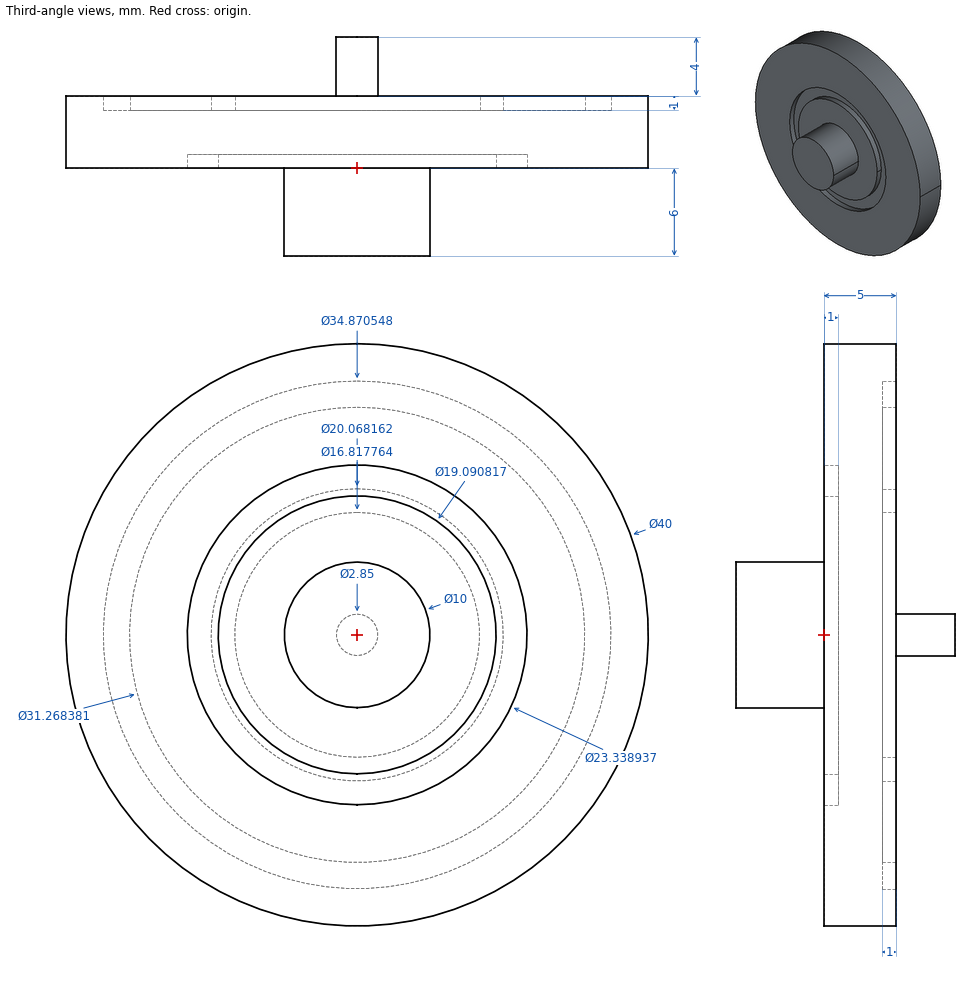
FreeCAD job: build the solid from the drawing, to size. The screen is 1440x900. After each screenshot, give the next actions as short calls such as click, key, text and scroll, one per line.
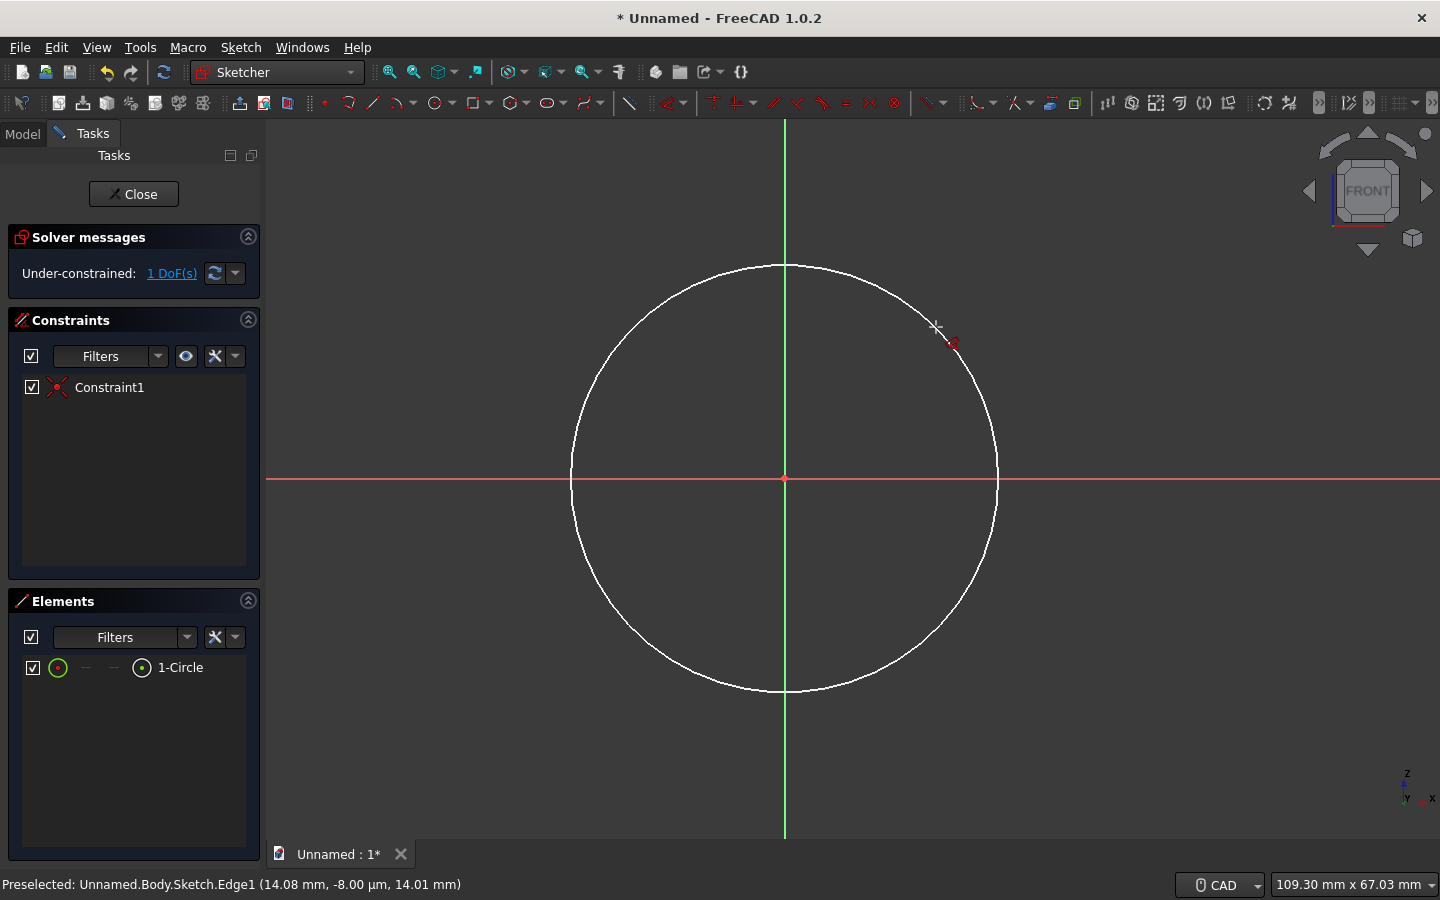
click(935, 327)
click(958, 304)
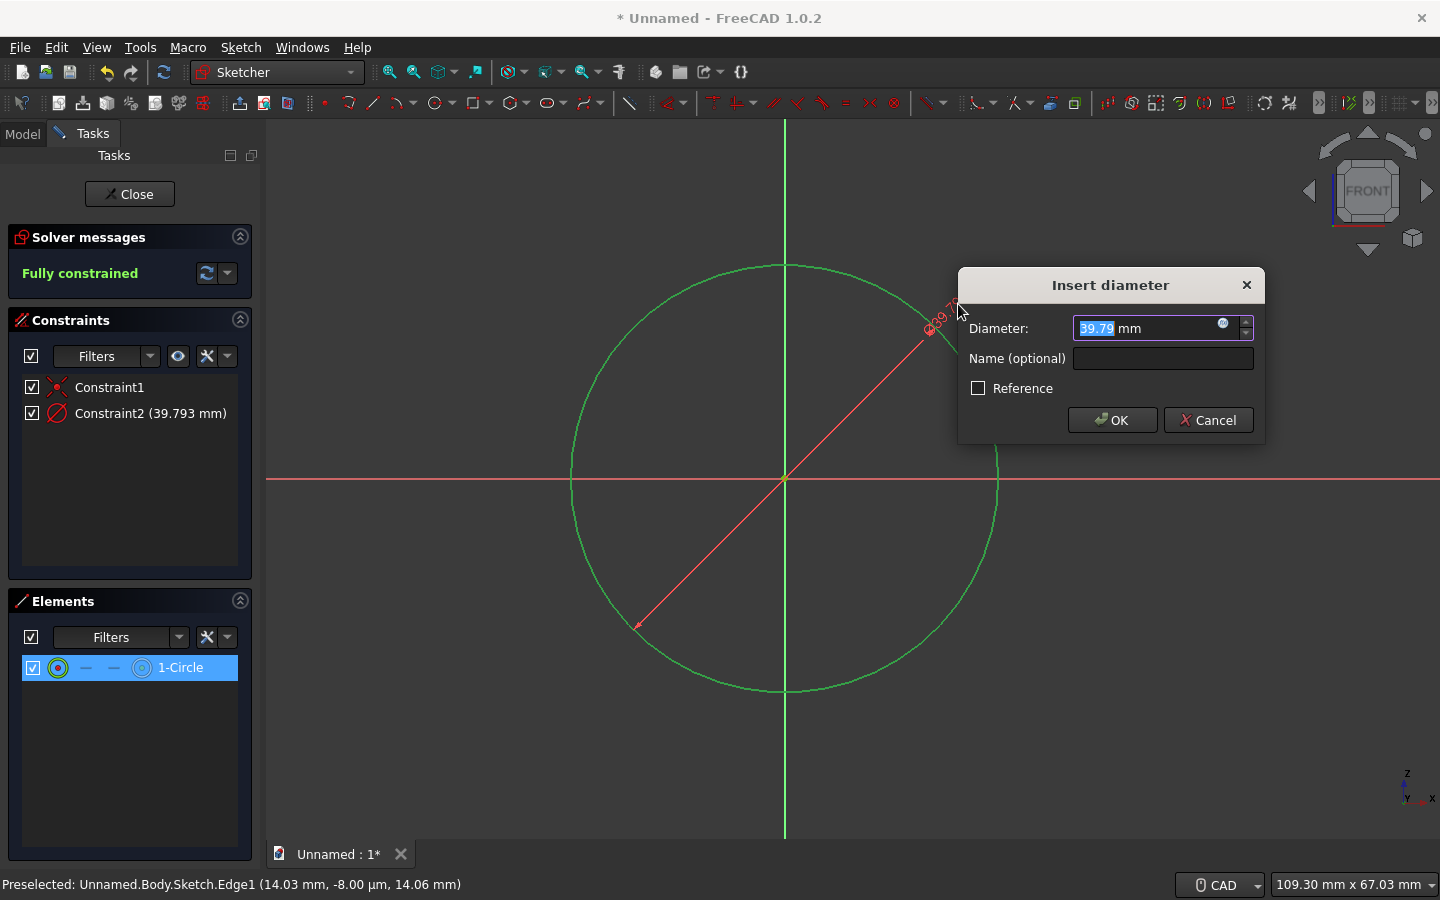
text(40)
key(Return)
key(Escape)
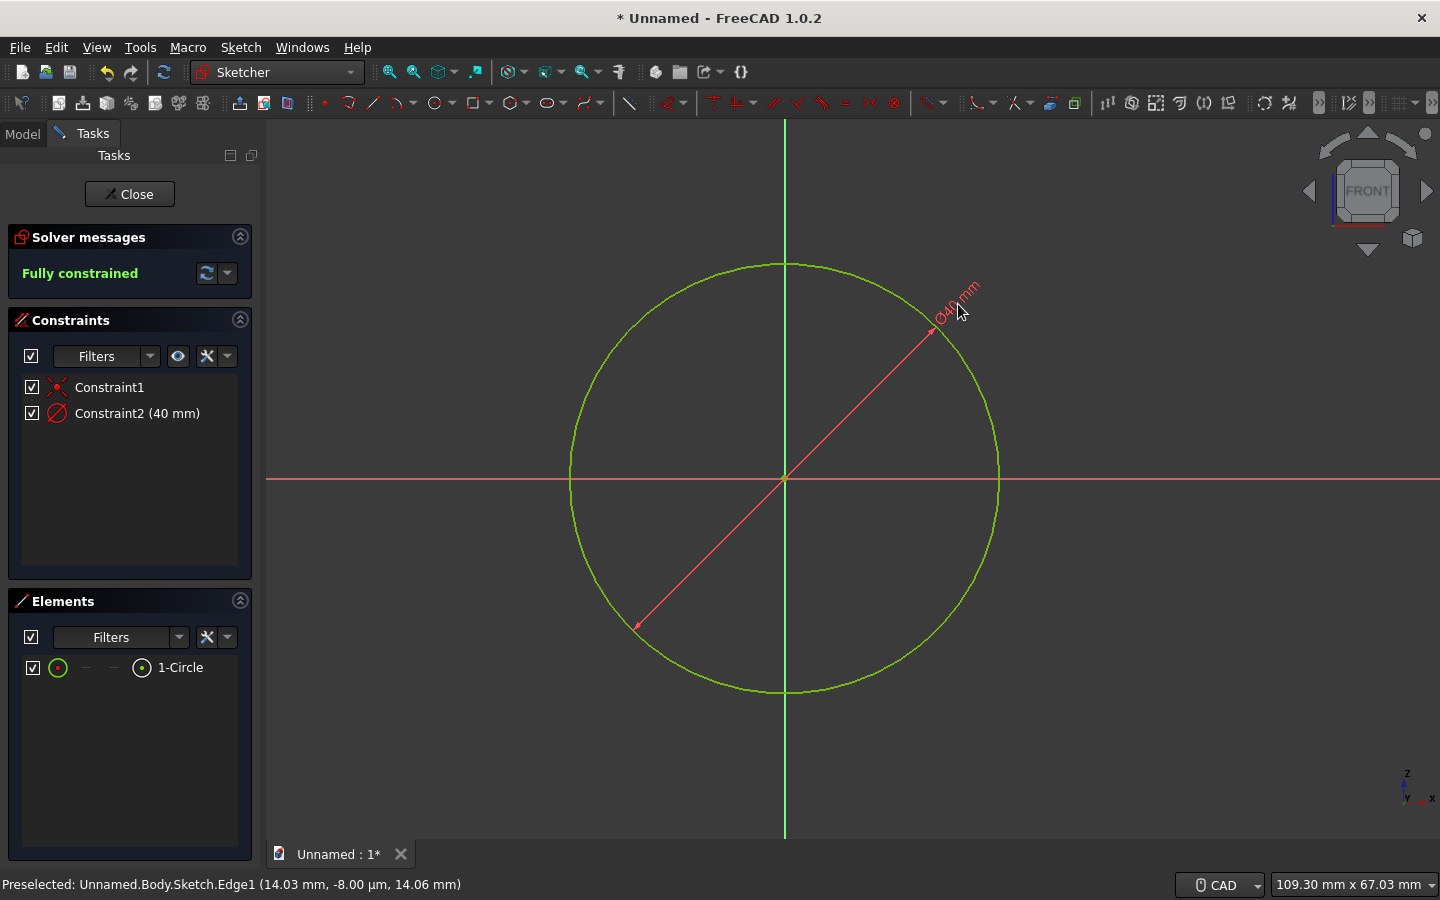
click(130, 194)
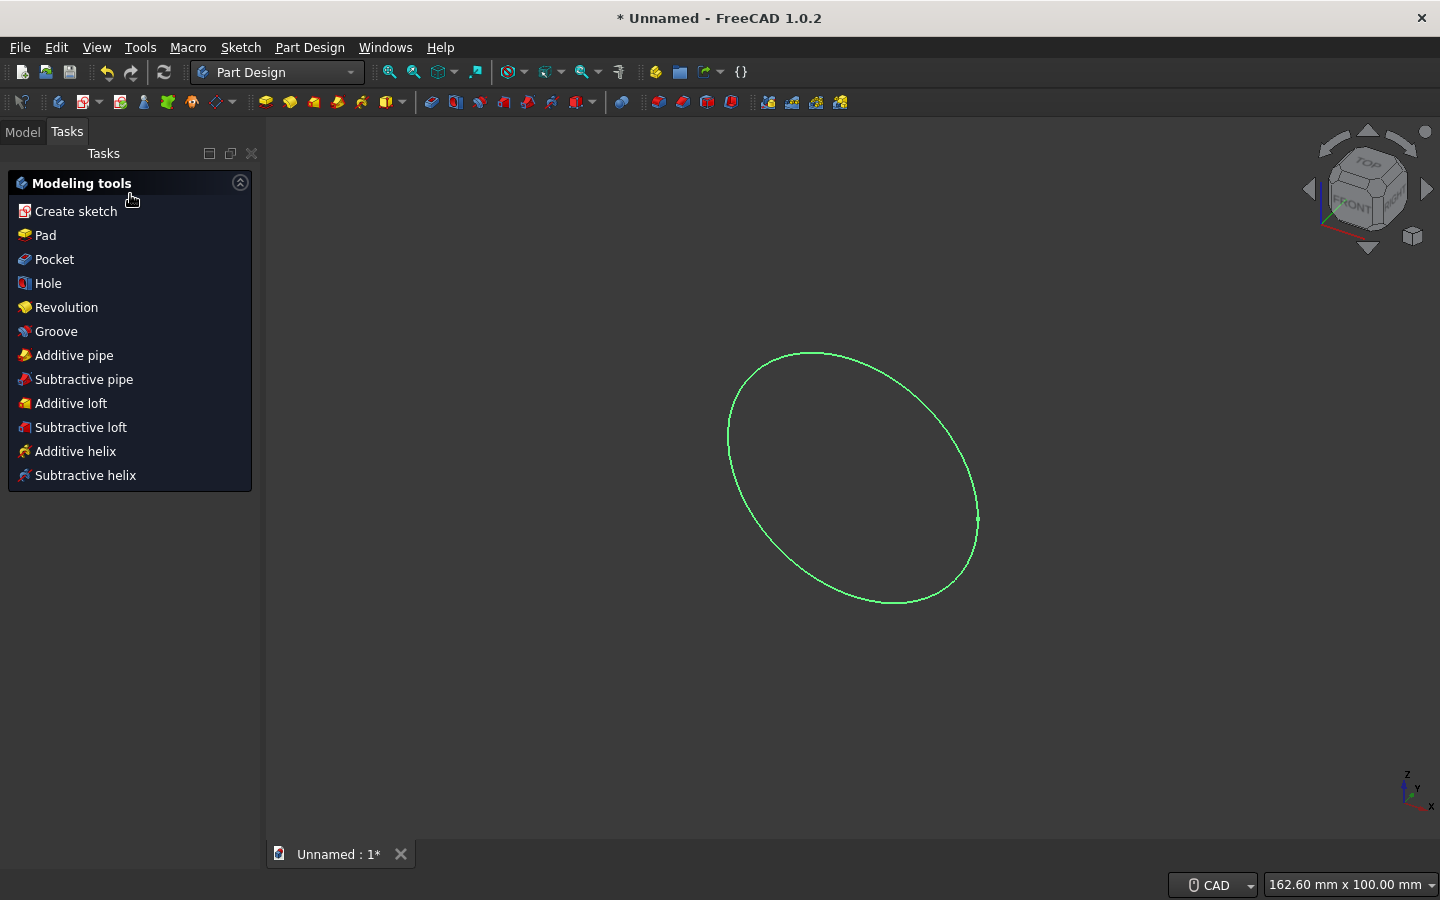
click(266, 102)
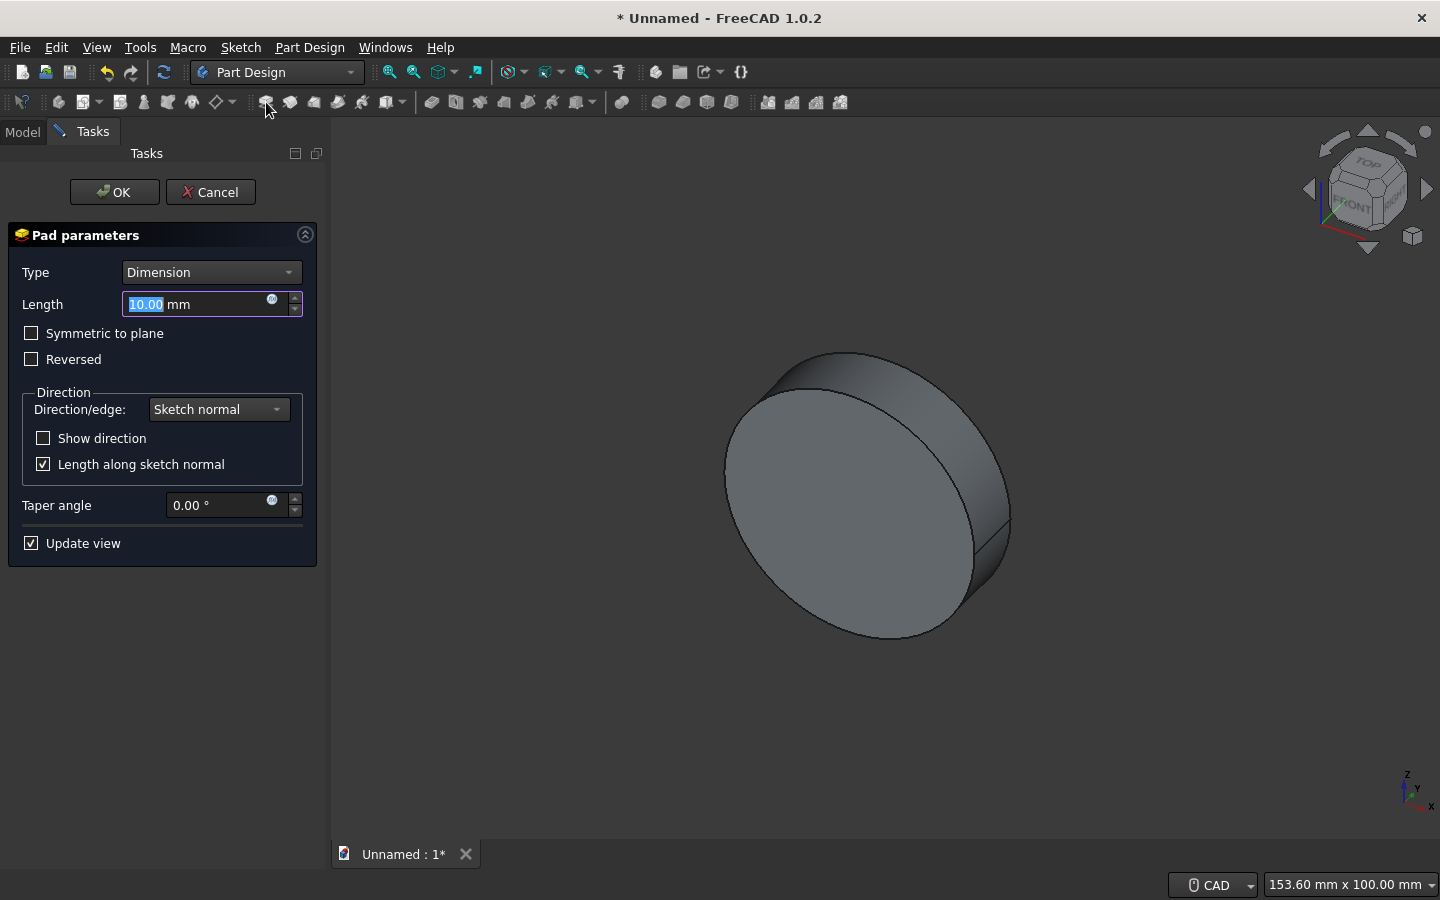
text(5)
key(Tab)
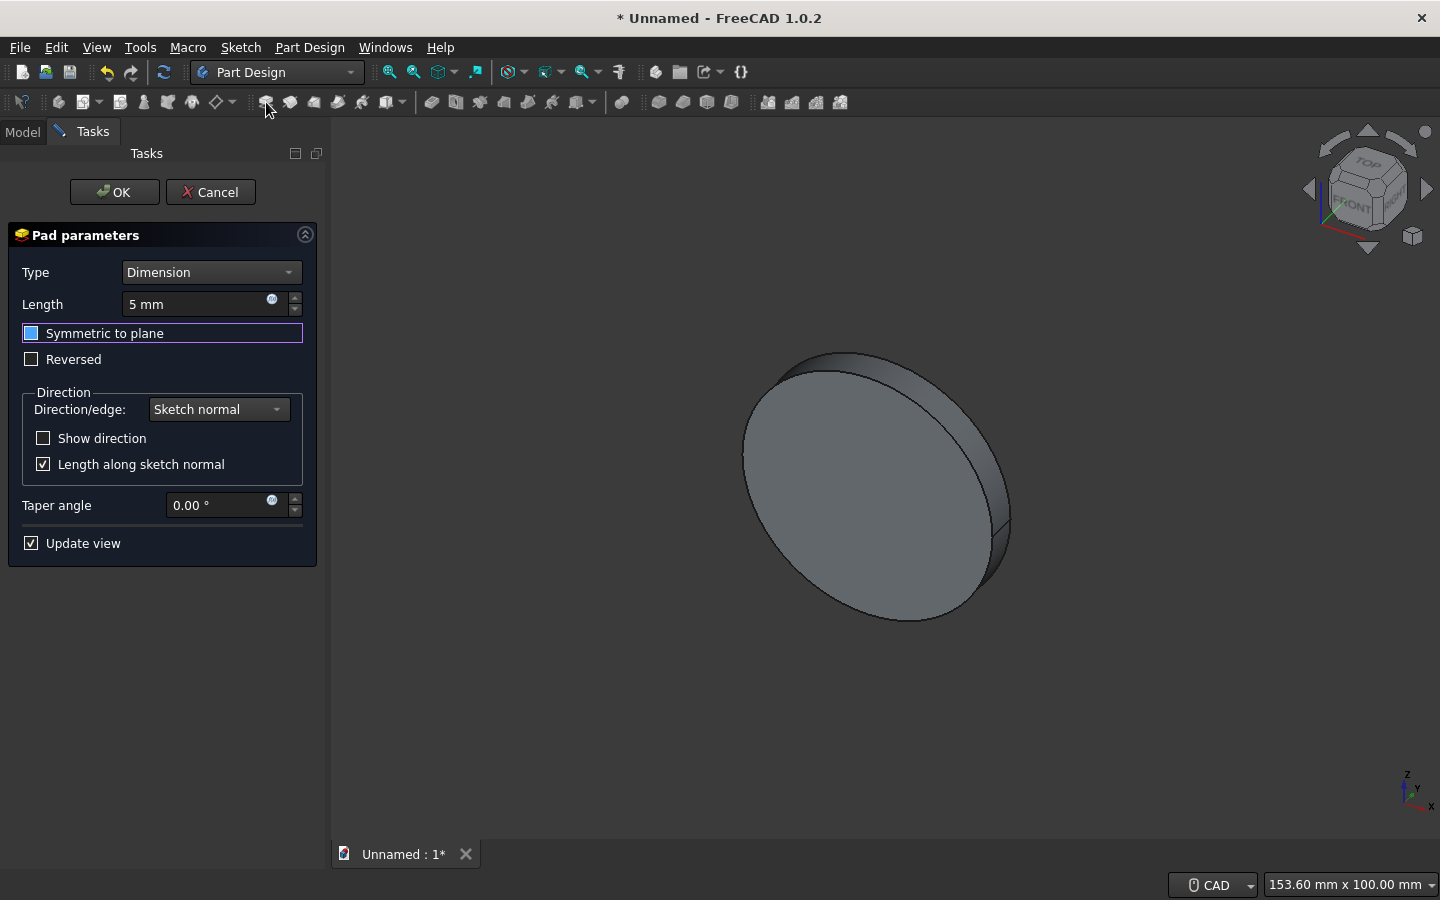
click(30, 359)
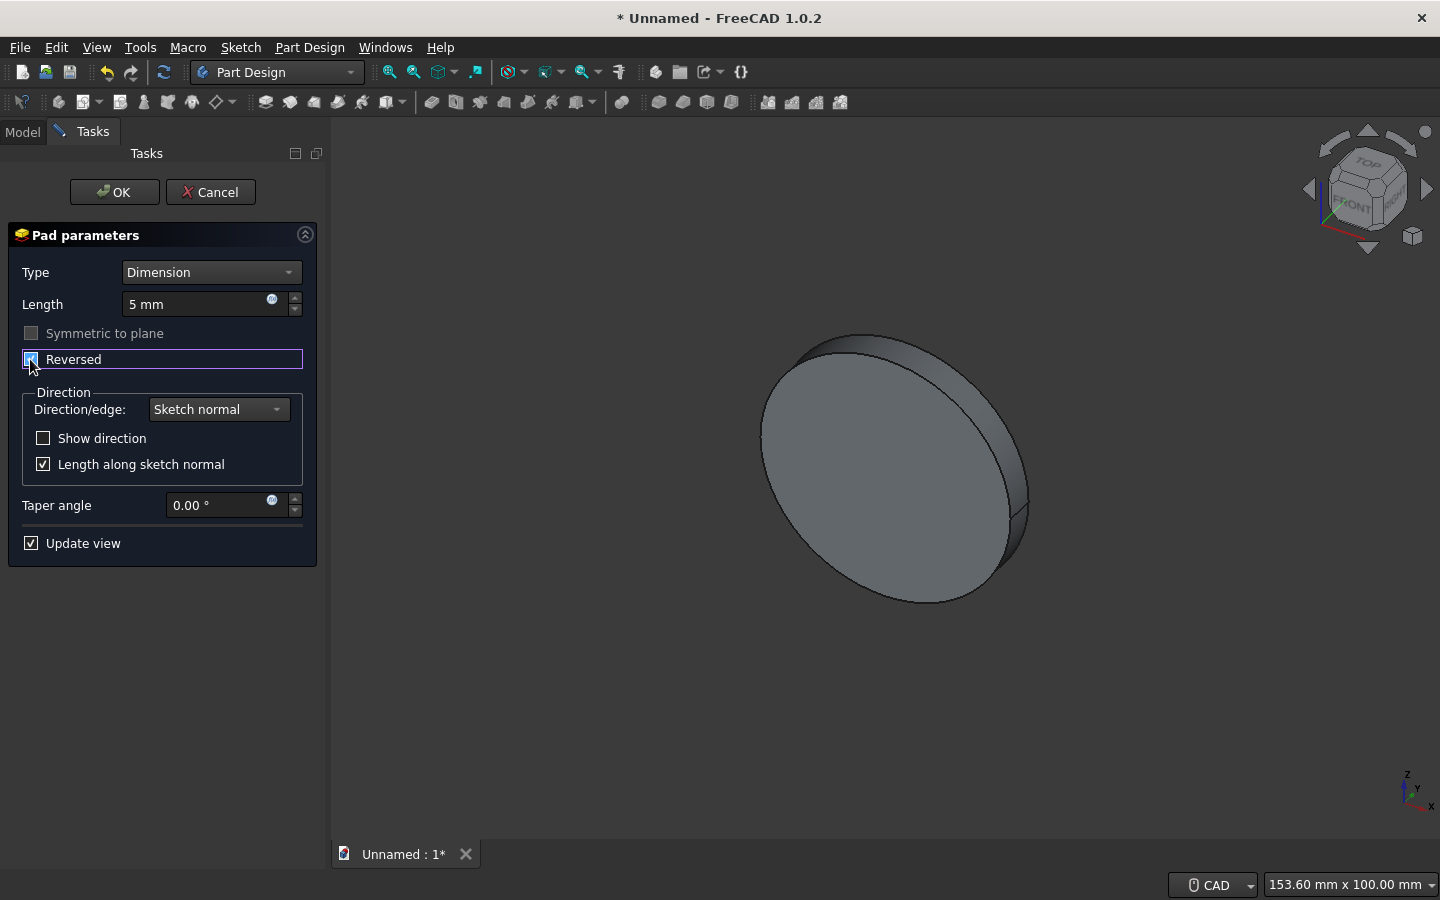
click(115, 192)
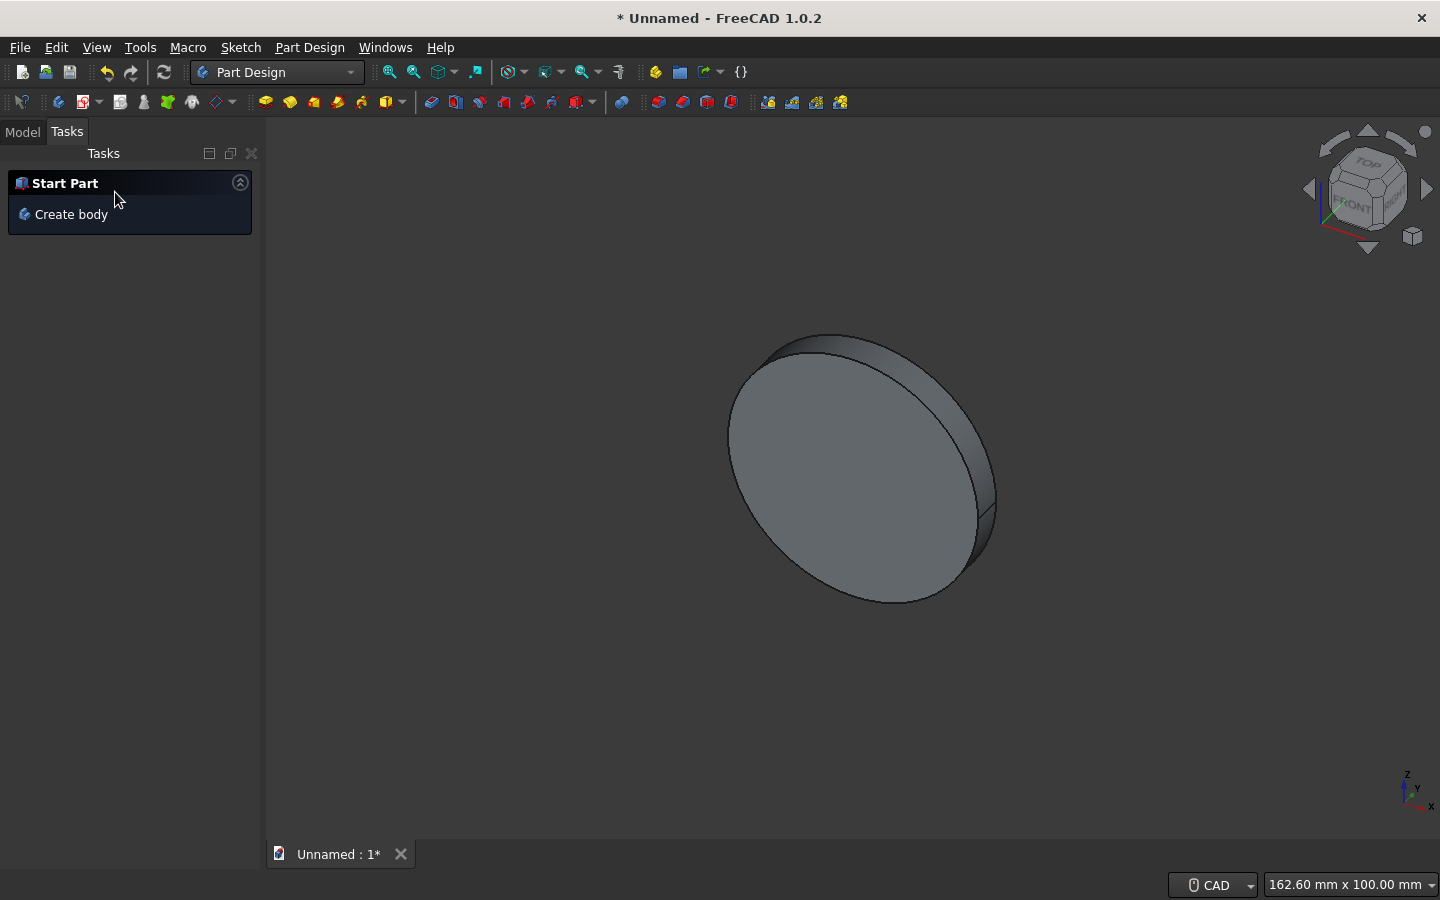
click(84, 102)